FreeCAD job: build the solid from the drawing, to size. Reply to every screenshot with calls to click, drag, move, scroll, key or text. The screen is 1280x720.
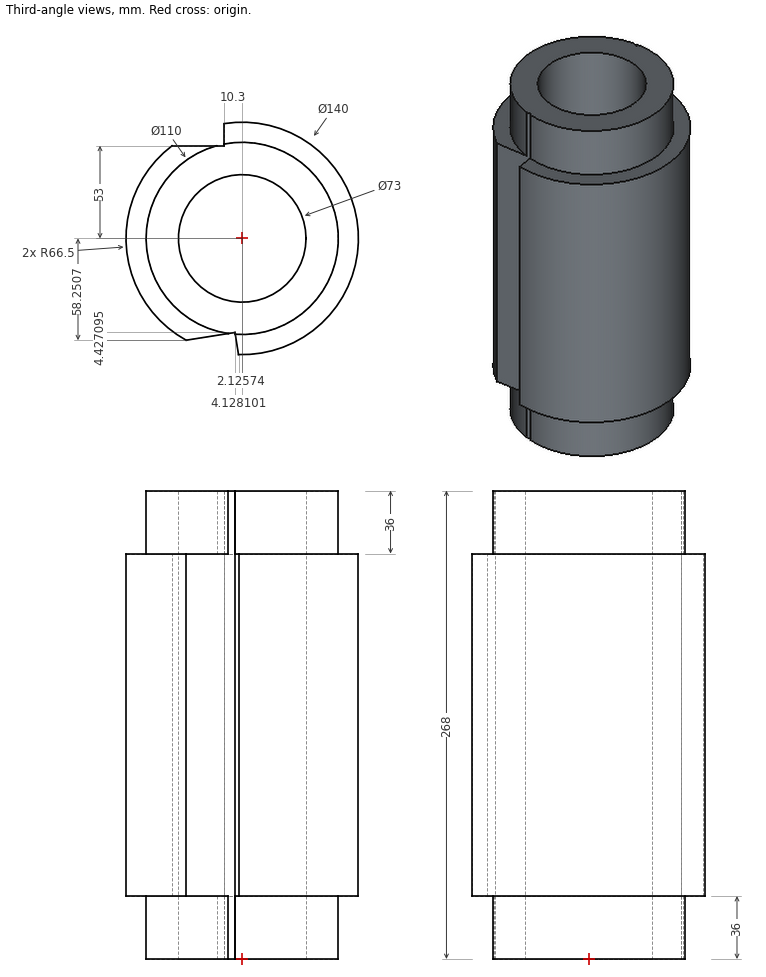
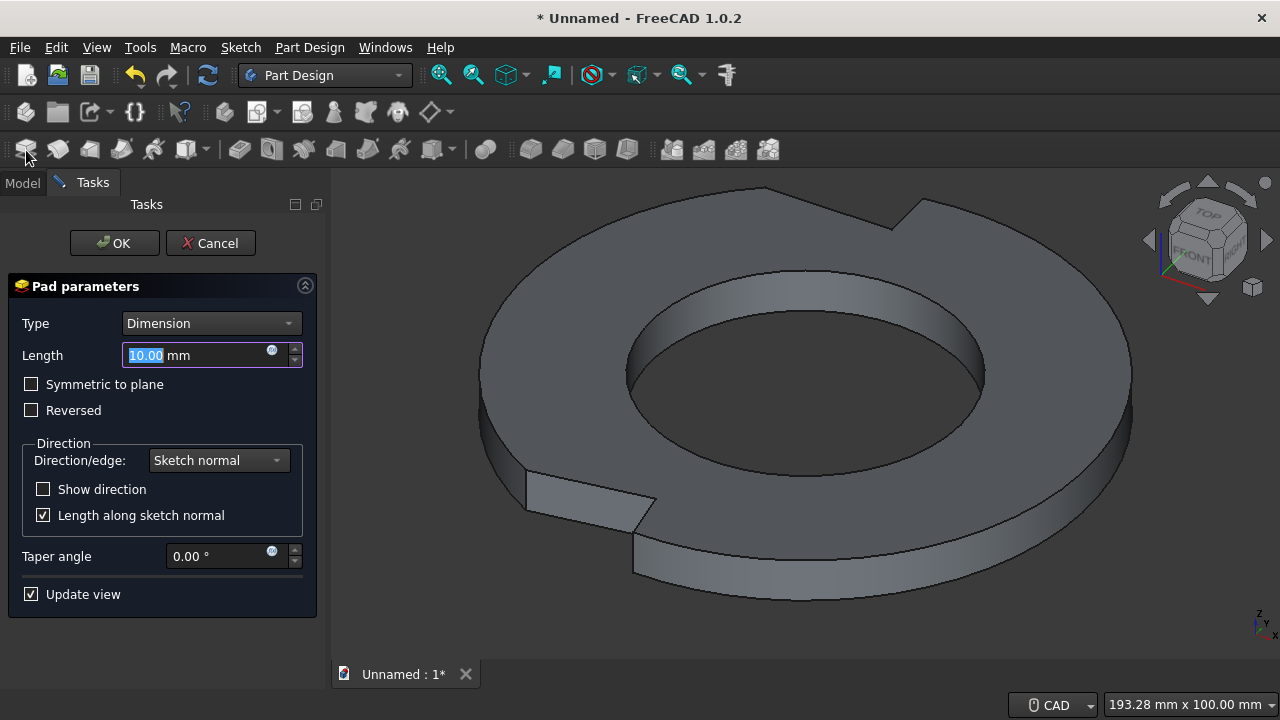
text(268)
key(Tab)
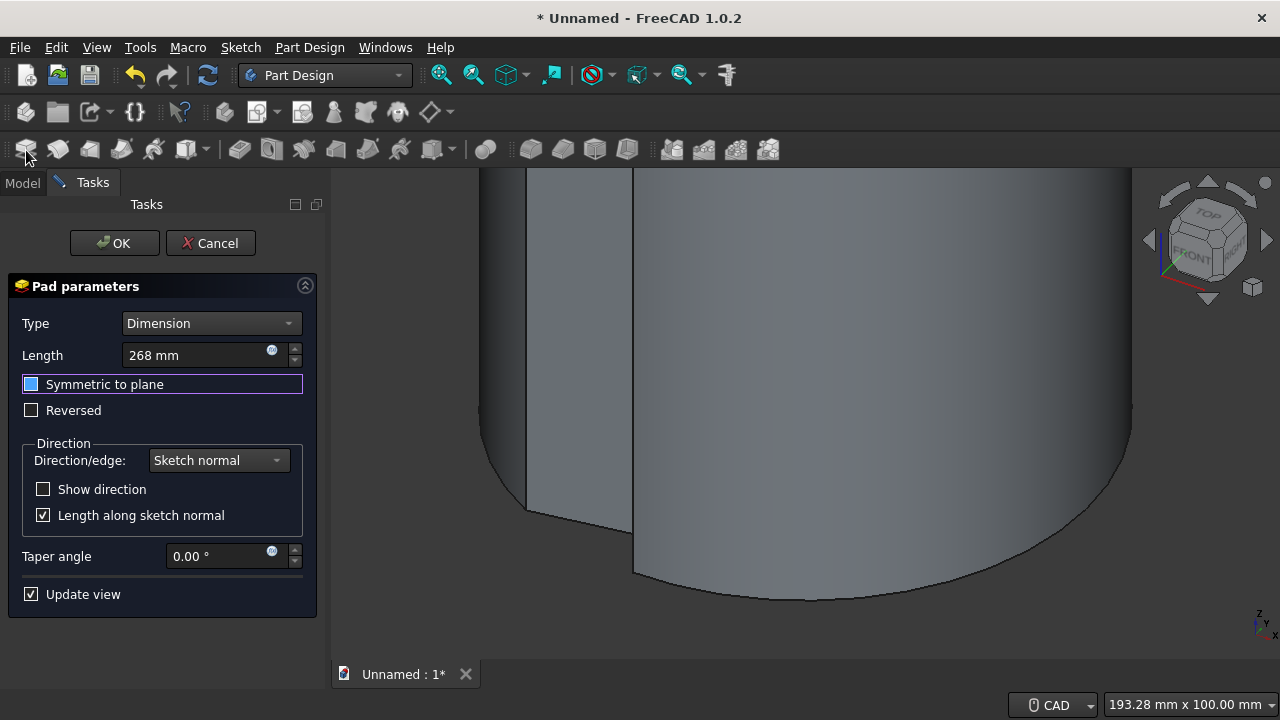
click(115, 243)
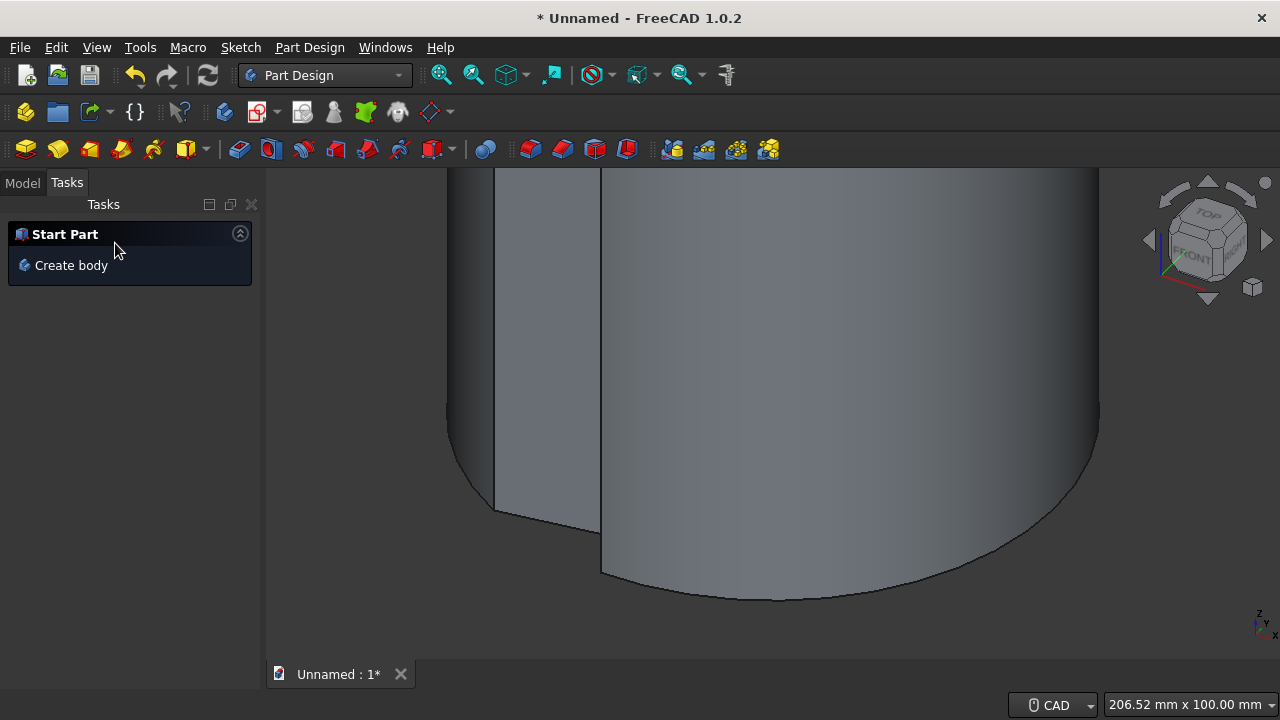
click(442, 76)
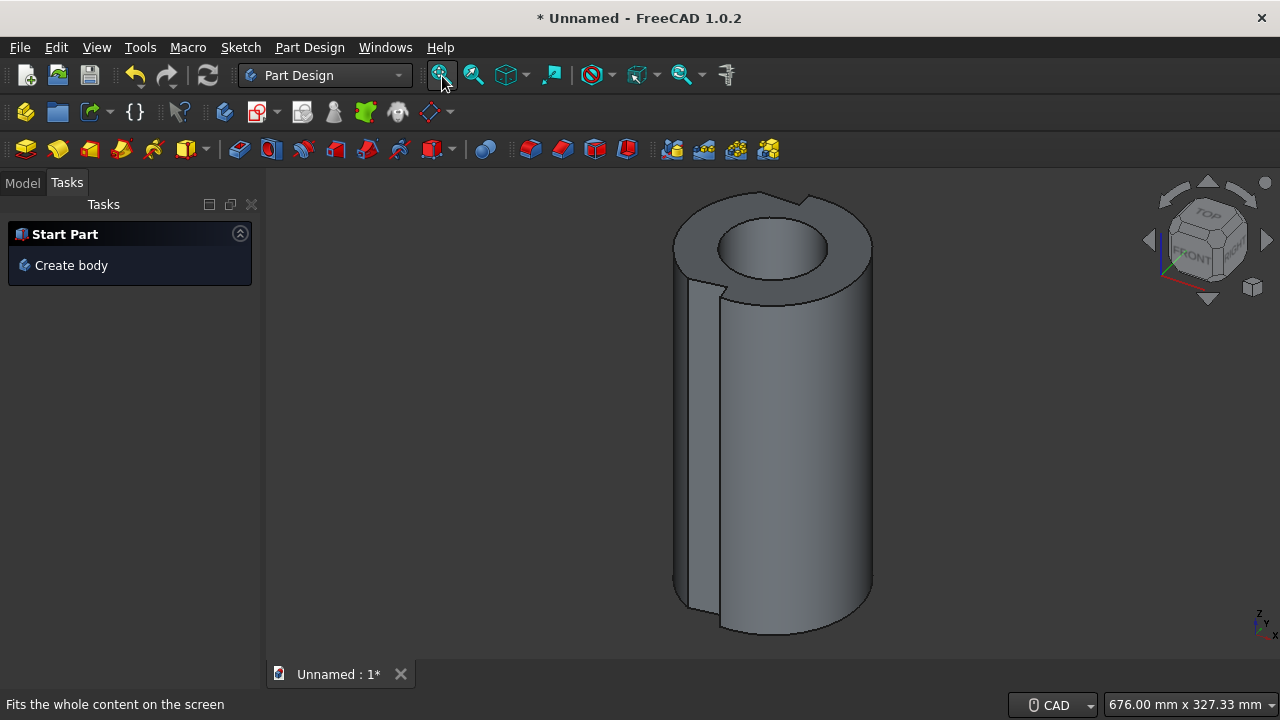
click(695, 260)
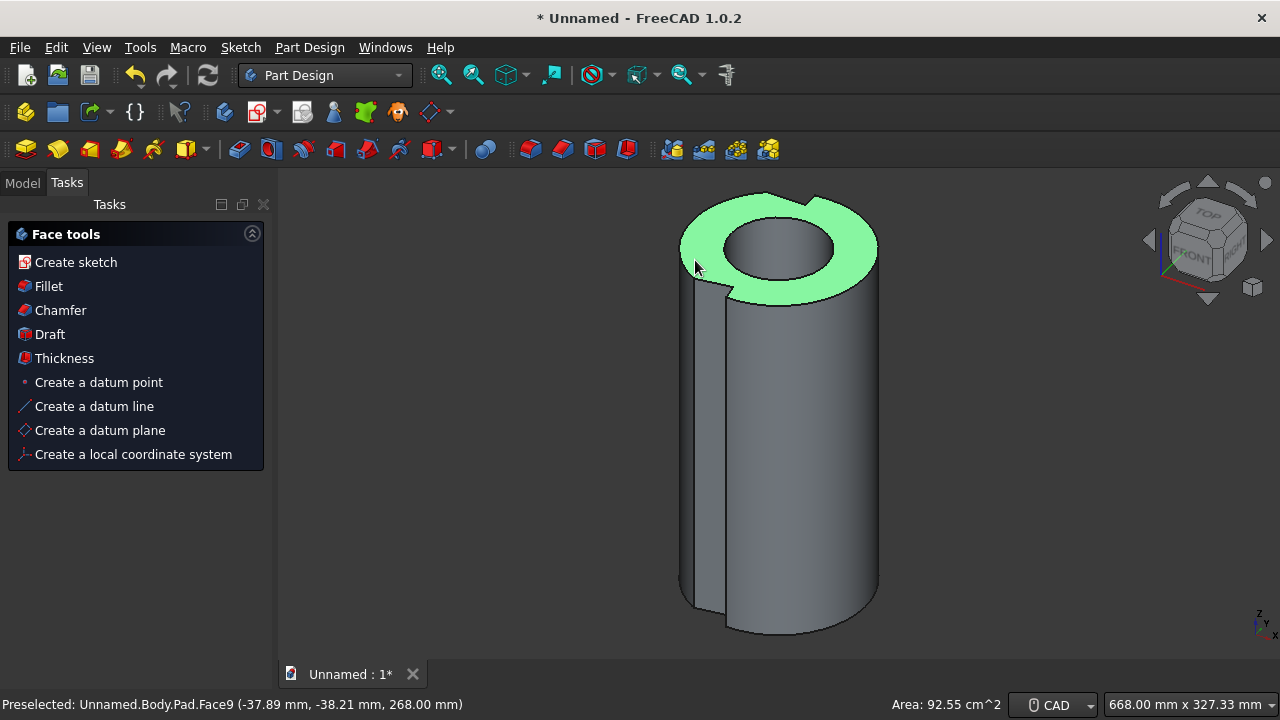
click(258, 112)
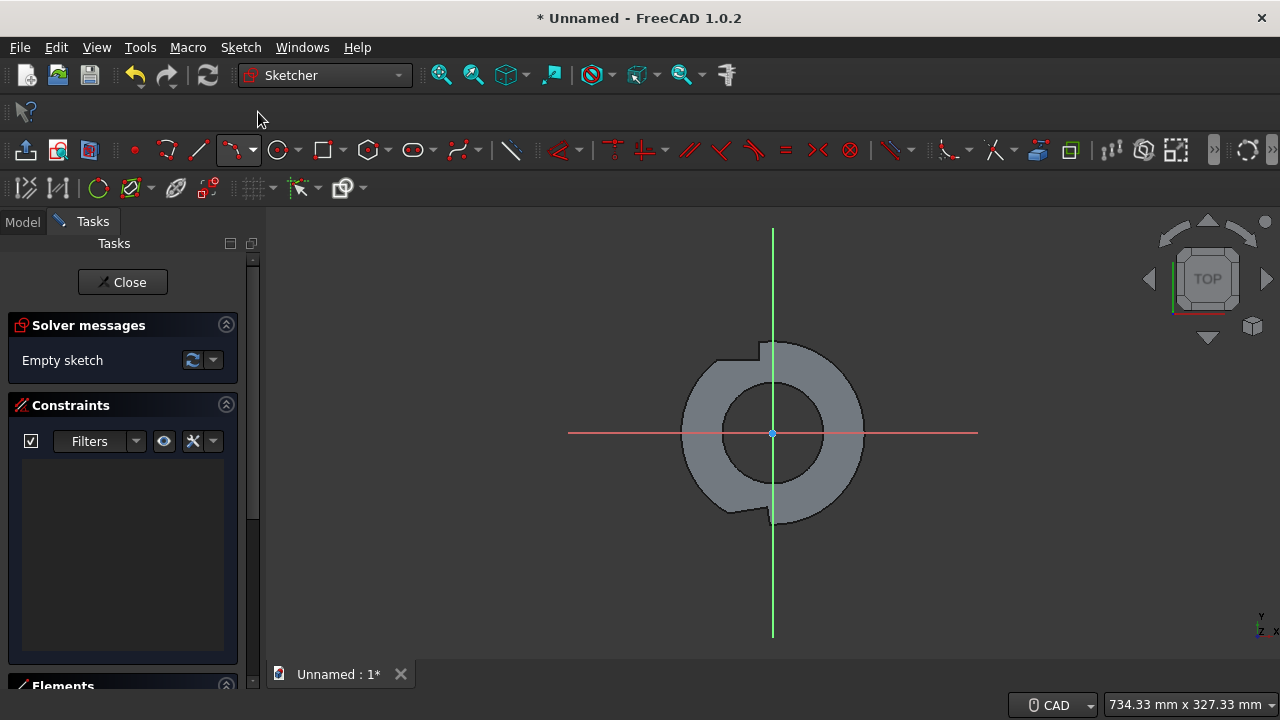
scroll(912, 433, up, 2)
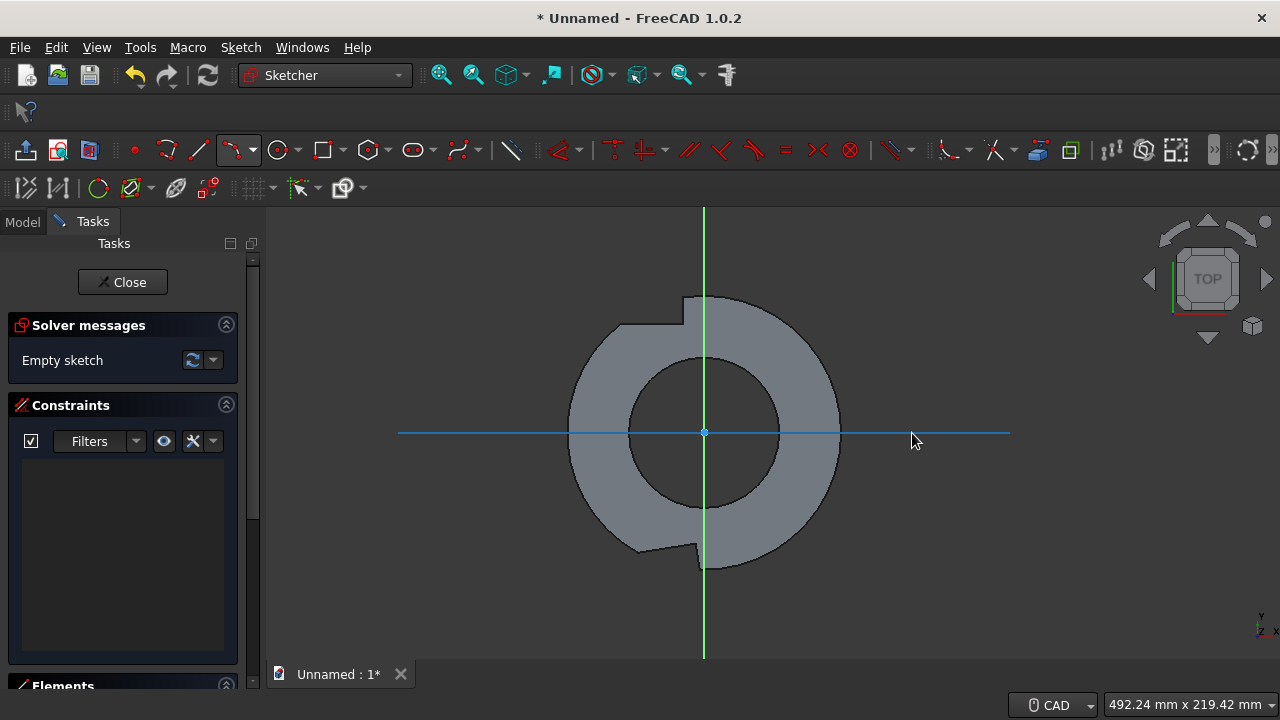
click(278, 150)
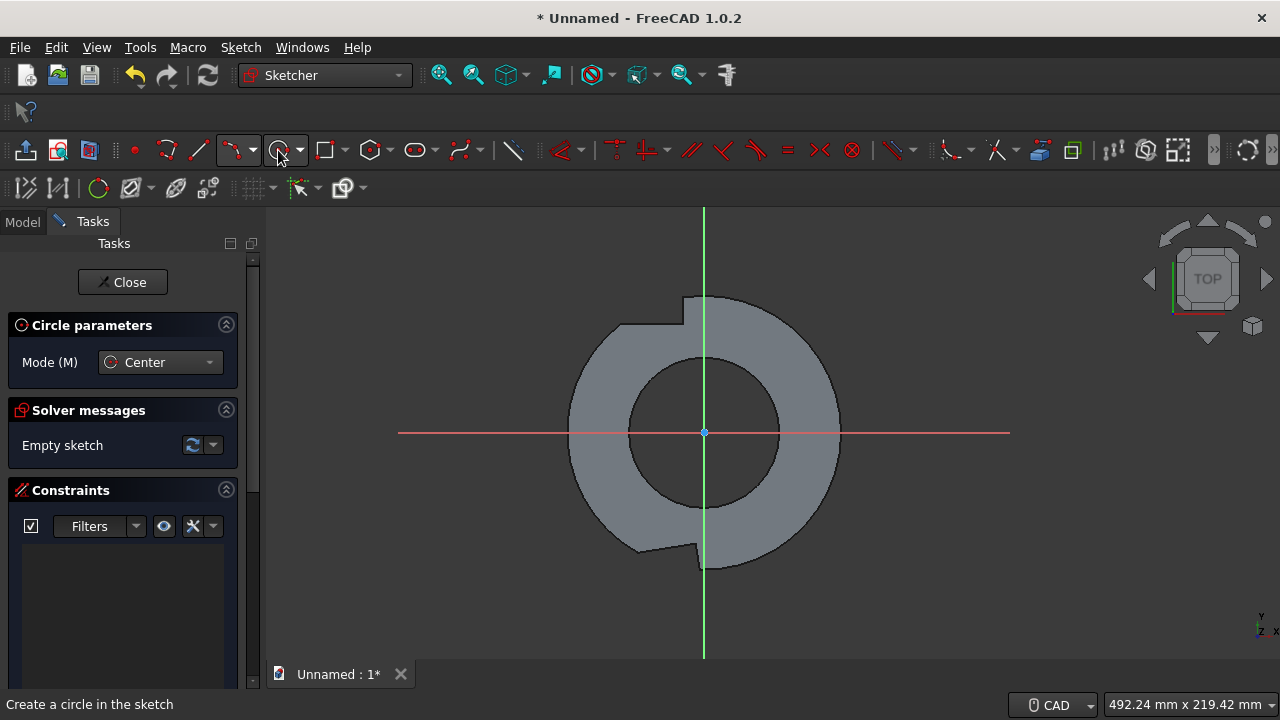
click(704, 433)
click(806, 331)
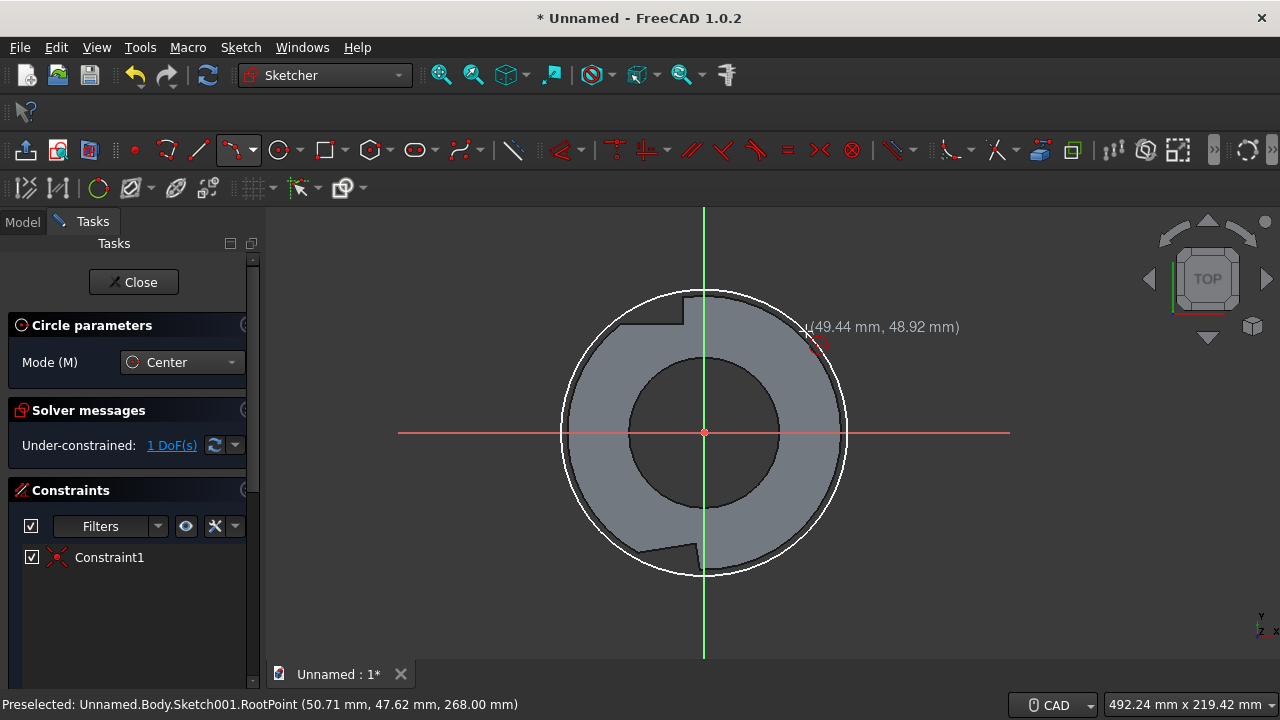
click(704, 433)
click(784, 353)
key(Escape)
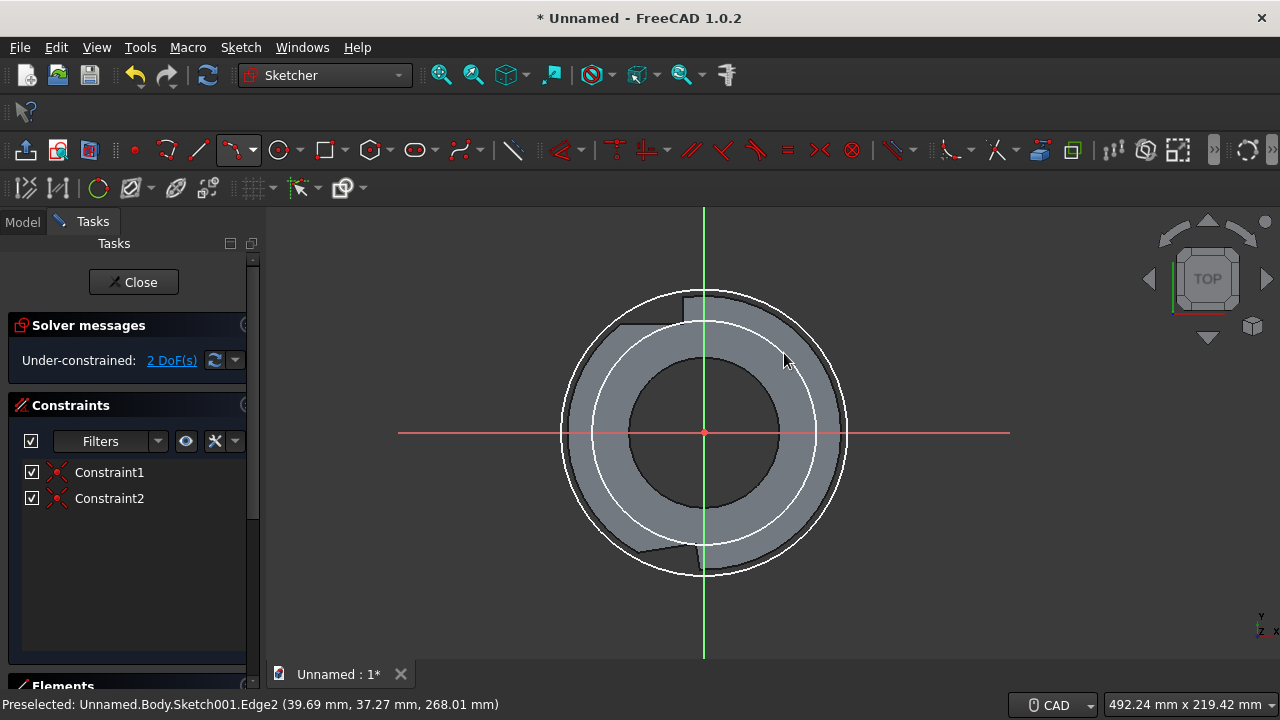
click(560, 150)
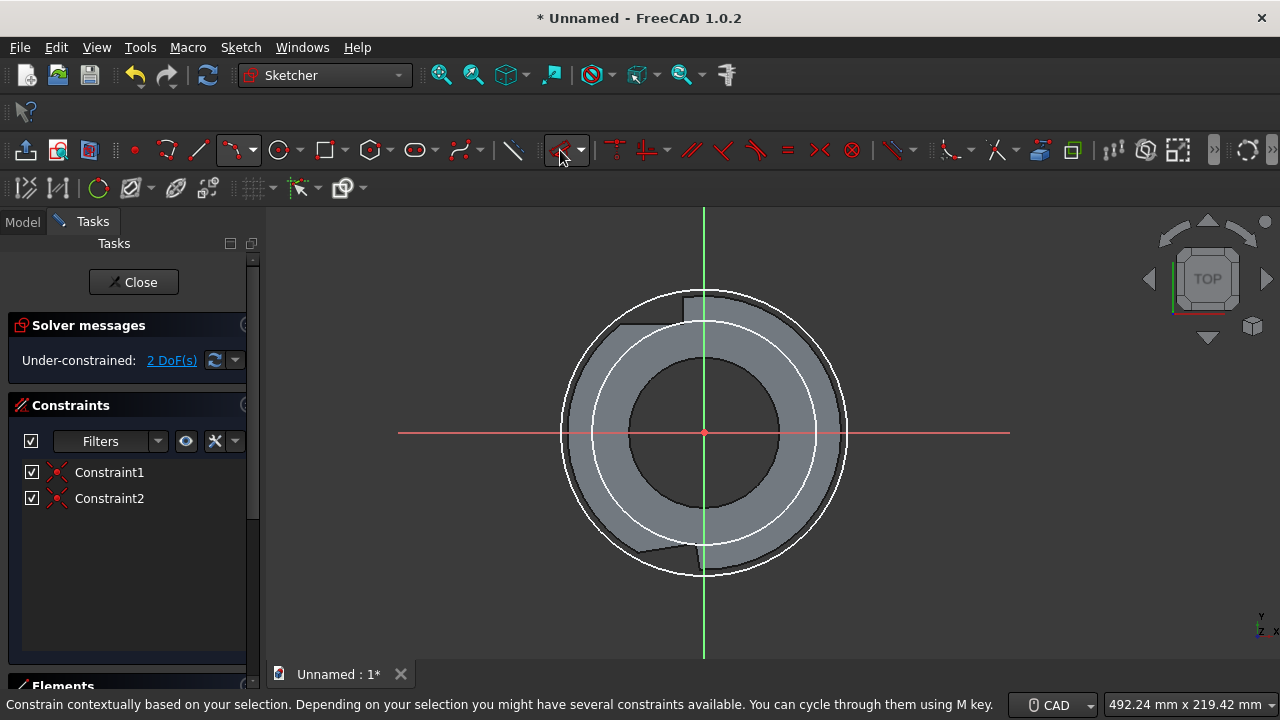
click(805, 331)
click(828, 308)